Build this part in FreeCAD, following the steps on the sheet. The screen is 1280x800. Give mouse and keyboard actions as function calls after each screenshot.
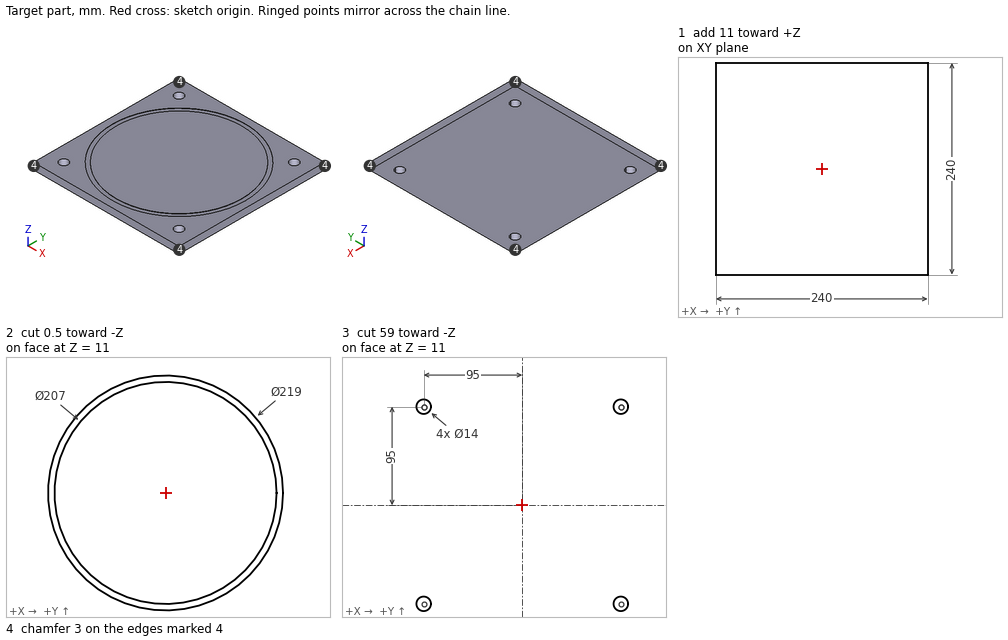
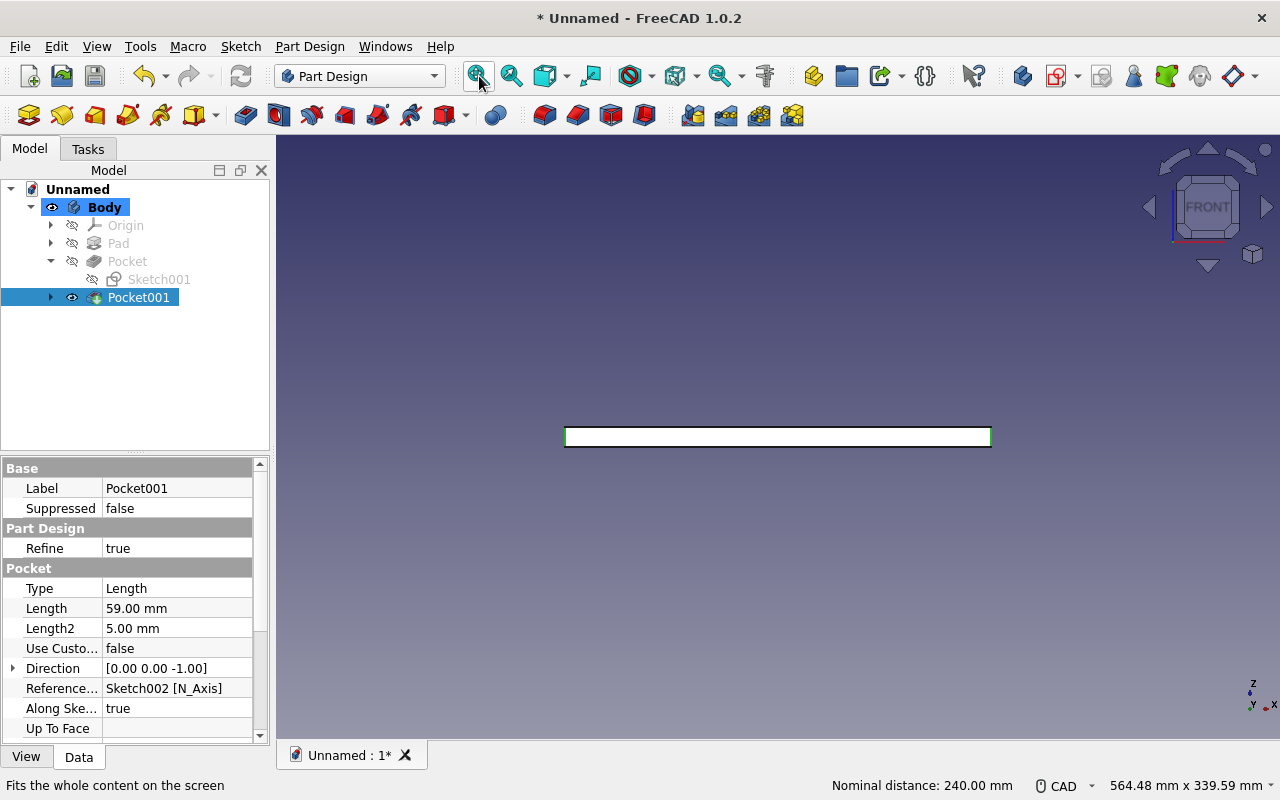
key(3)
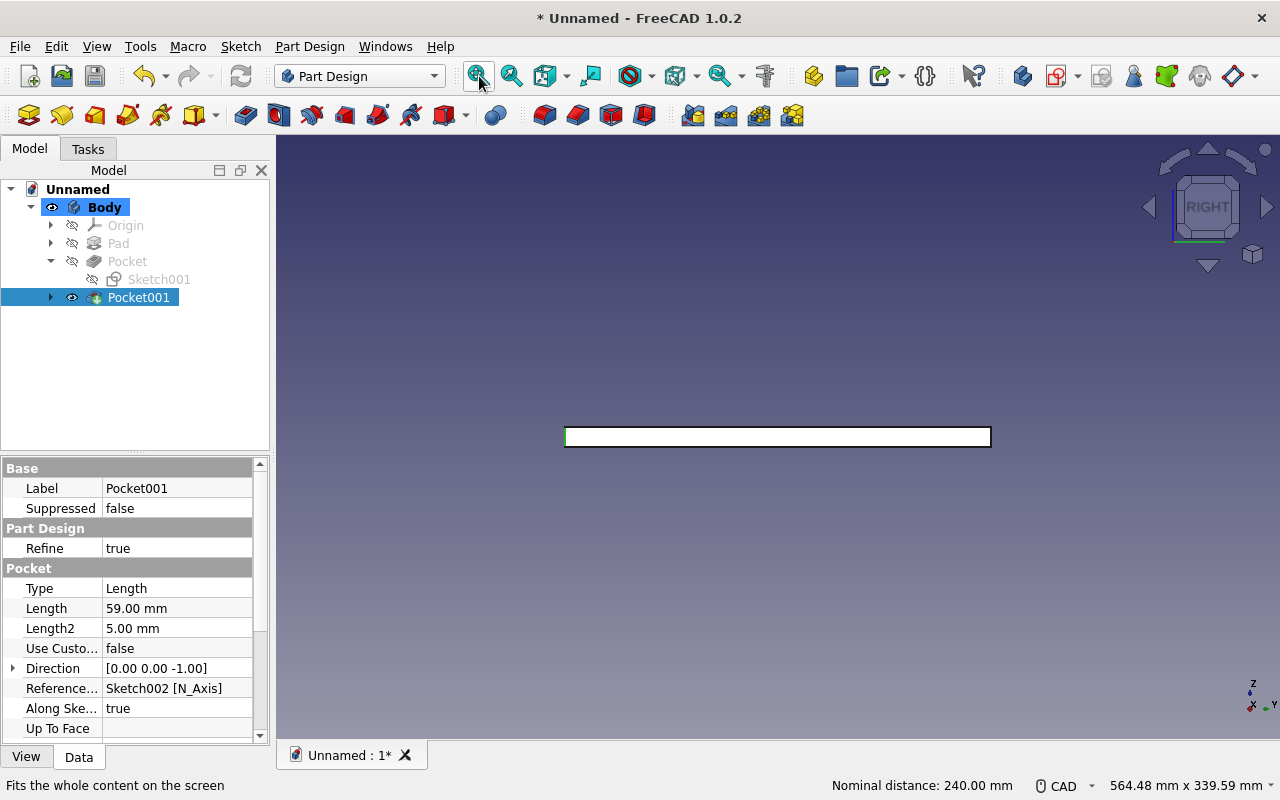
click(479, 76)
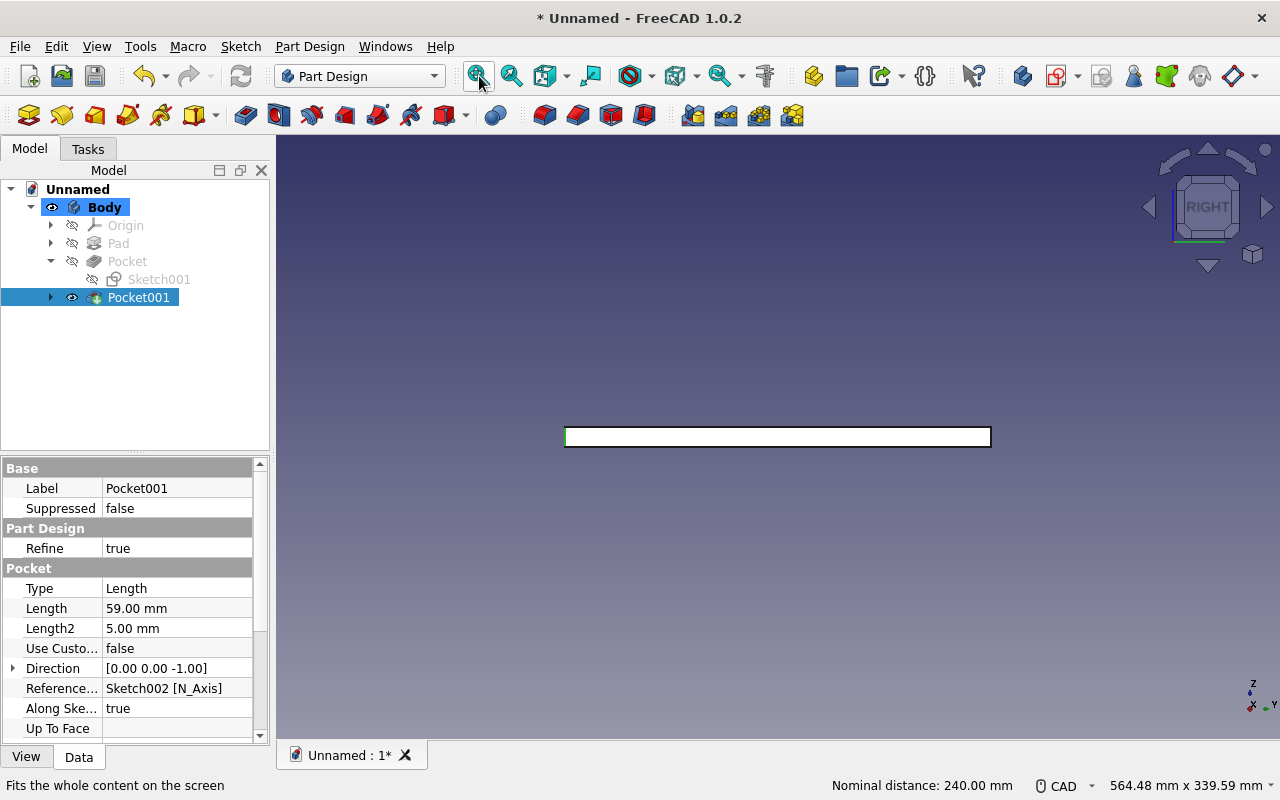
click(991, 436, ctrl)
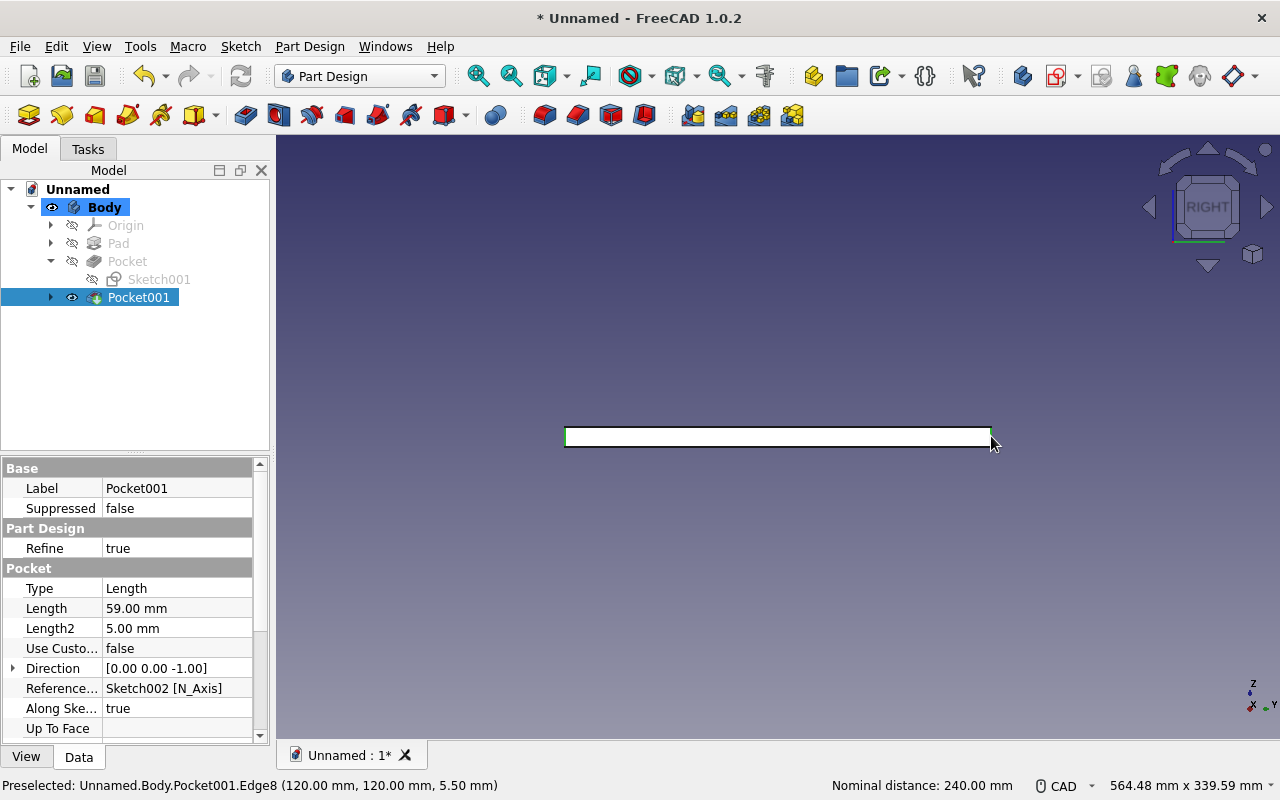
scroll(991, 436, up, 4)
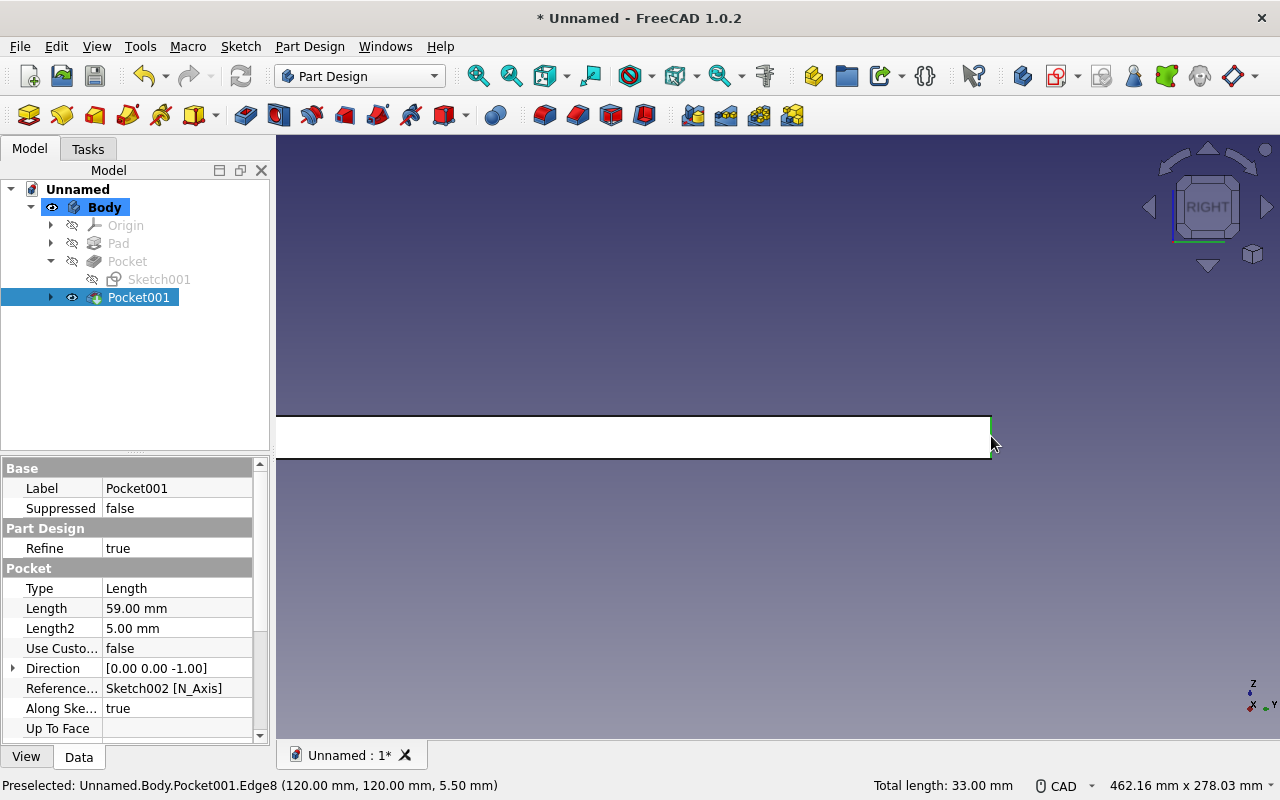
click(479, 76)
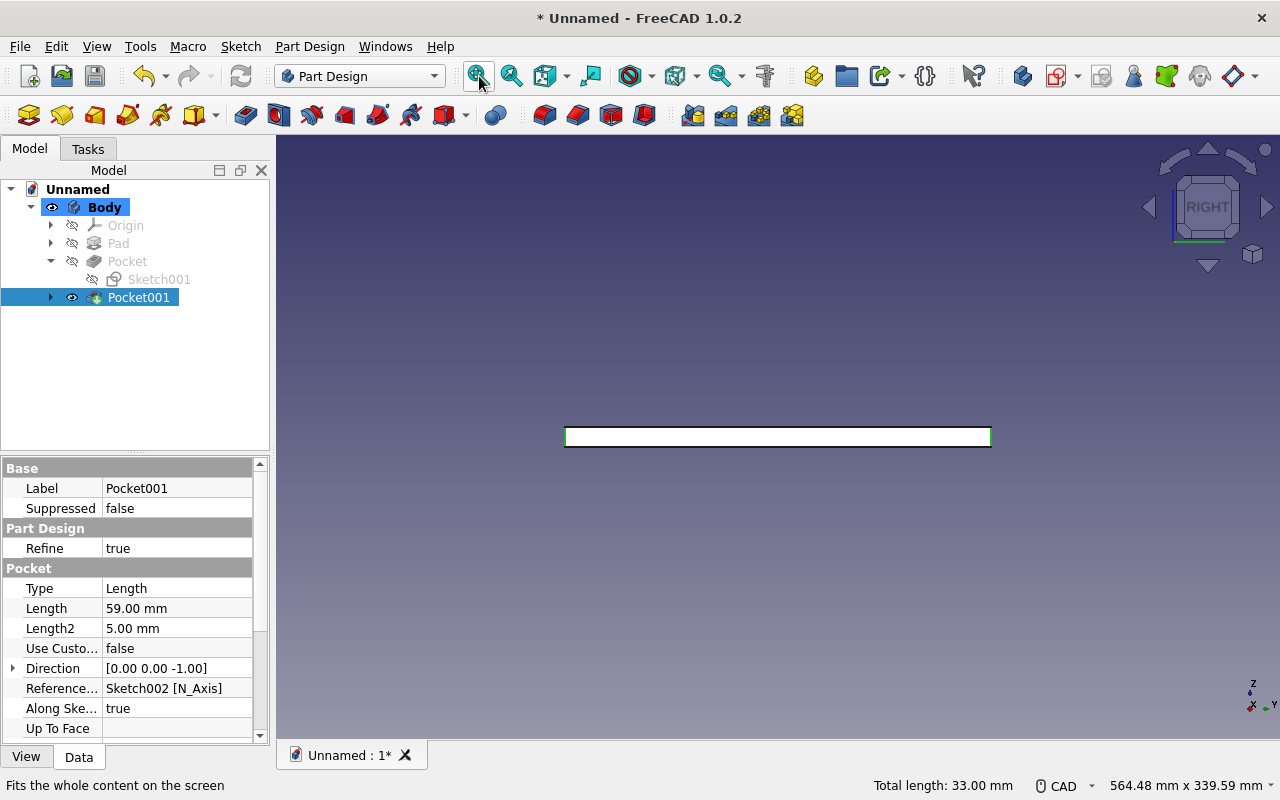
key(5)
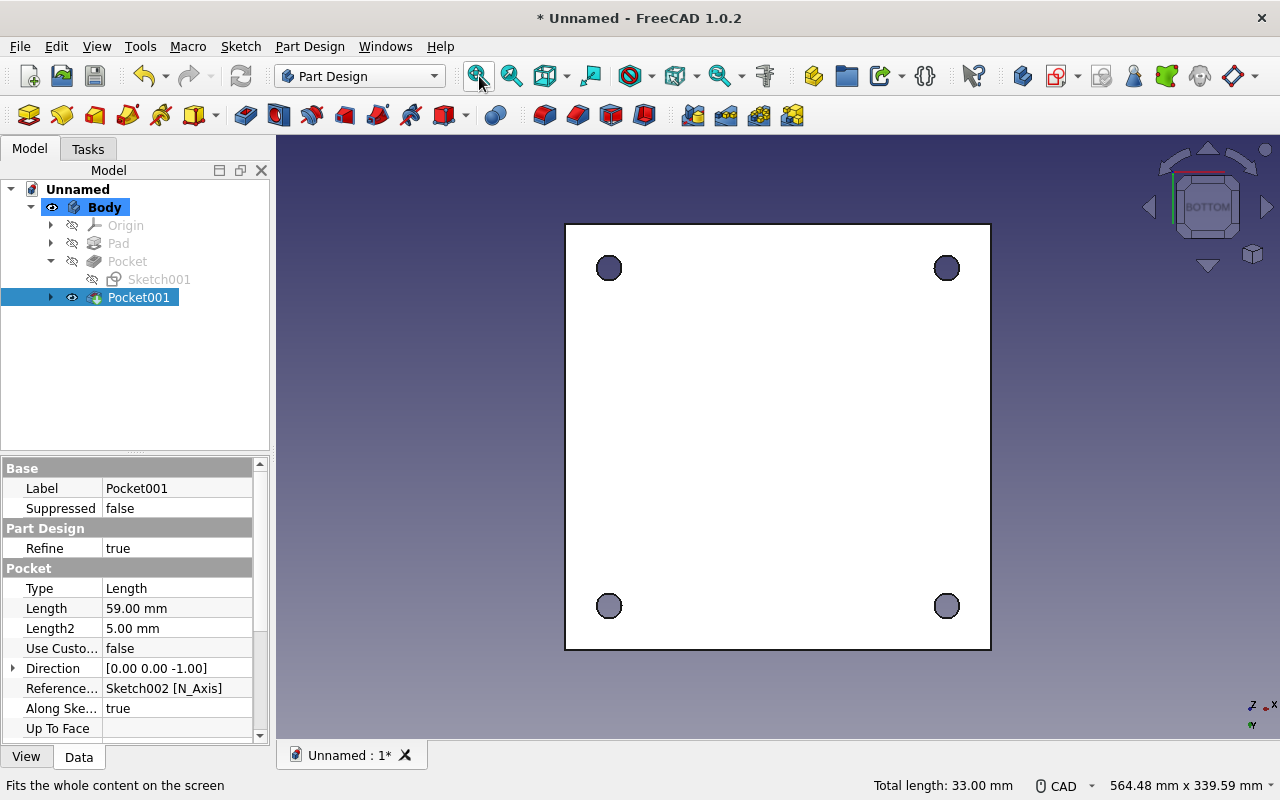
scroll(565, 649, up, 4)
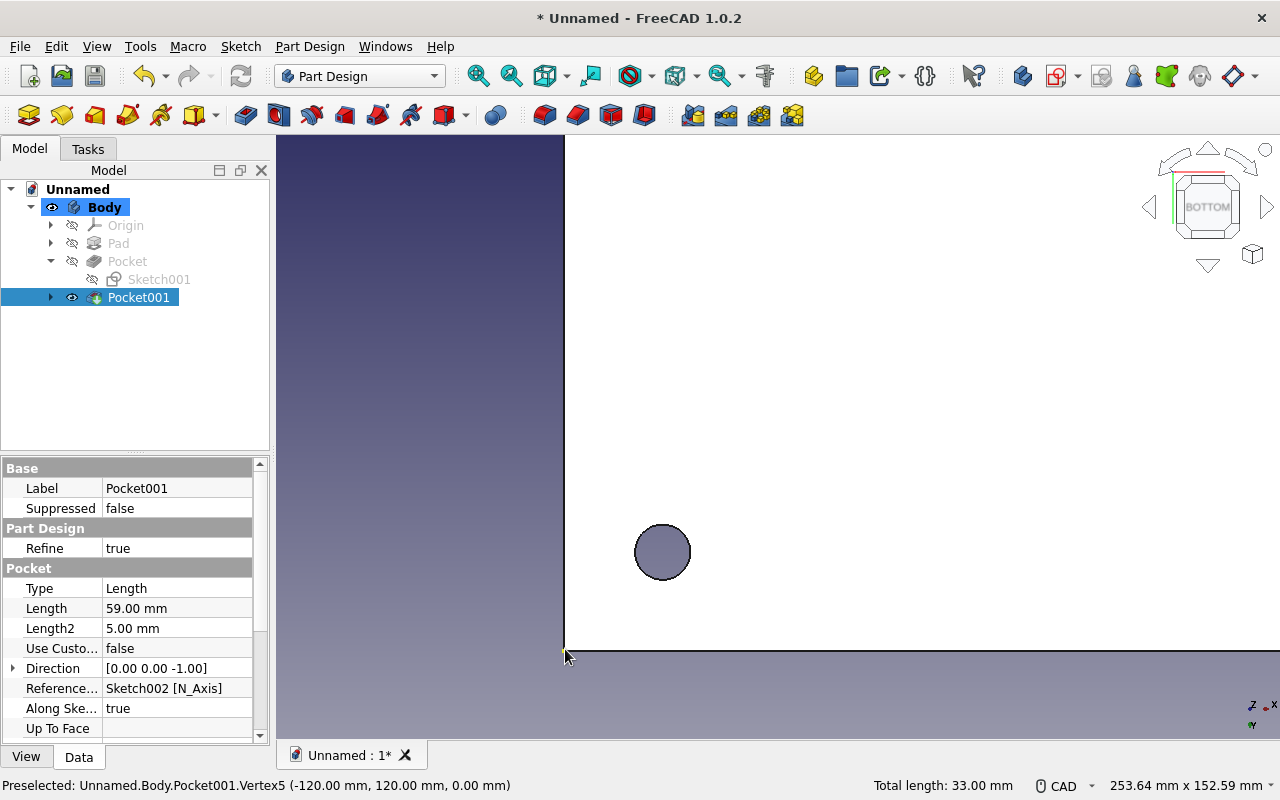
click(479, 76)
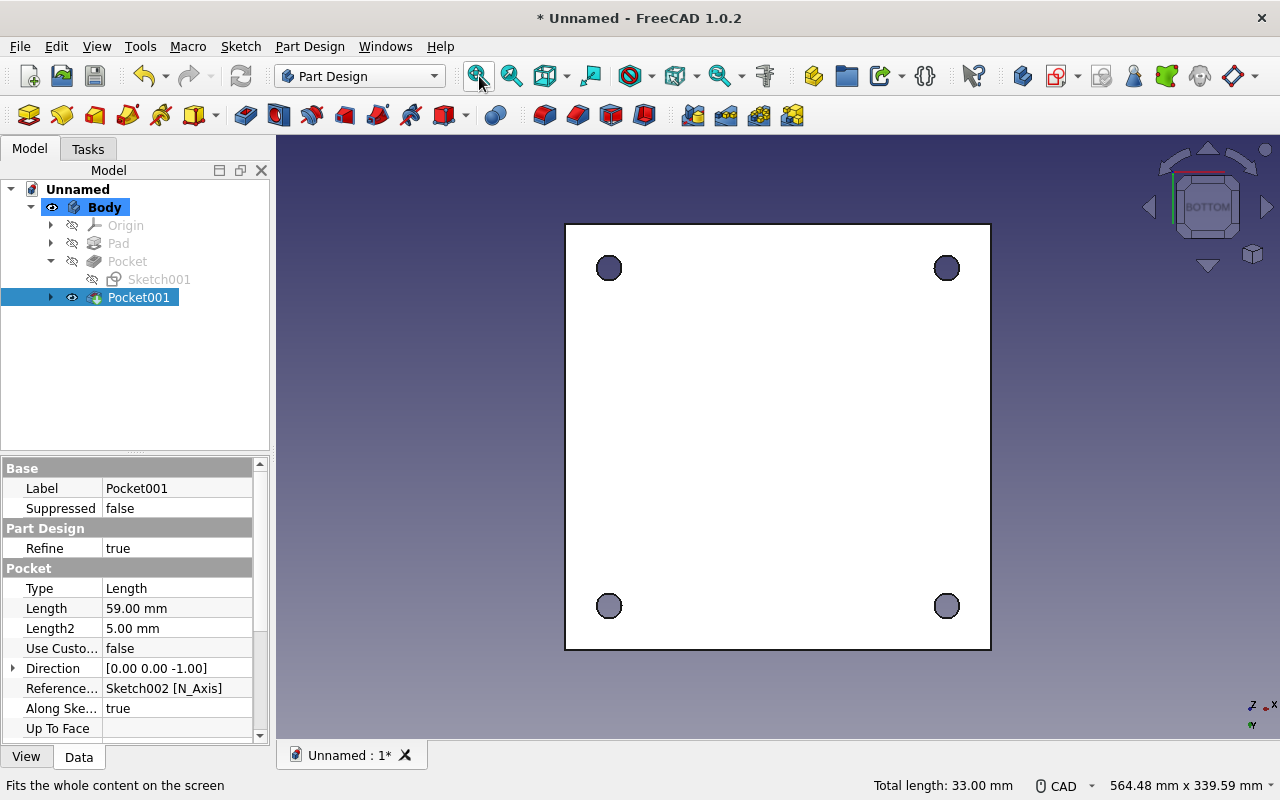
key(4)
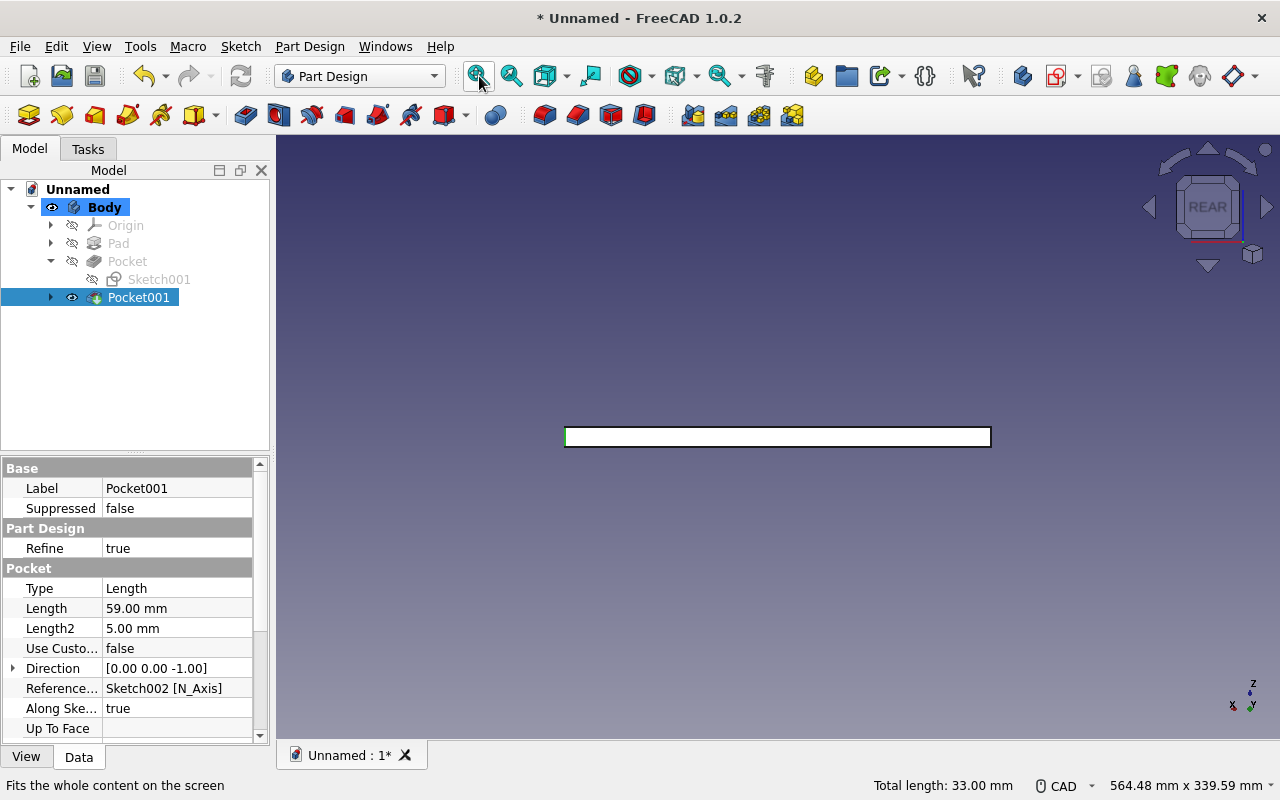
click(479, 76)